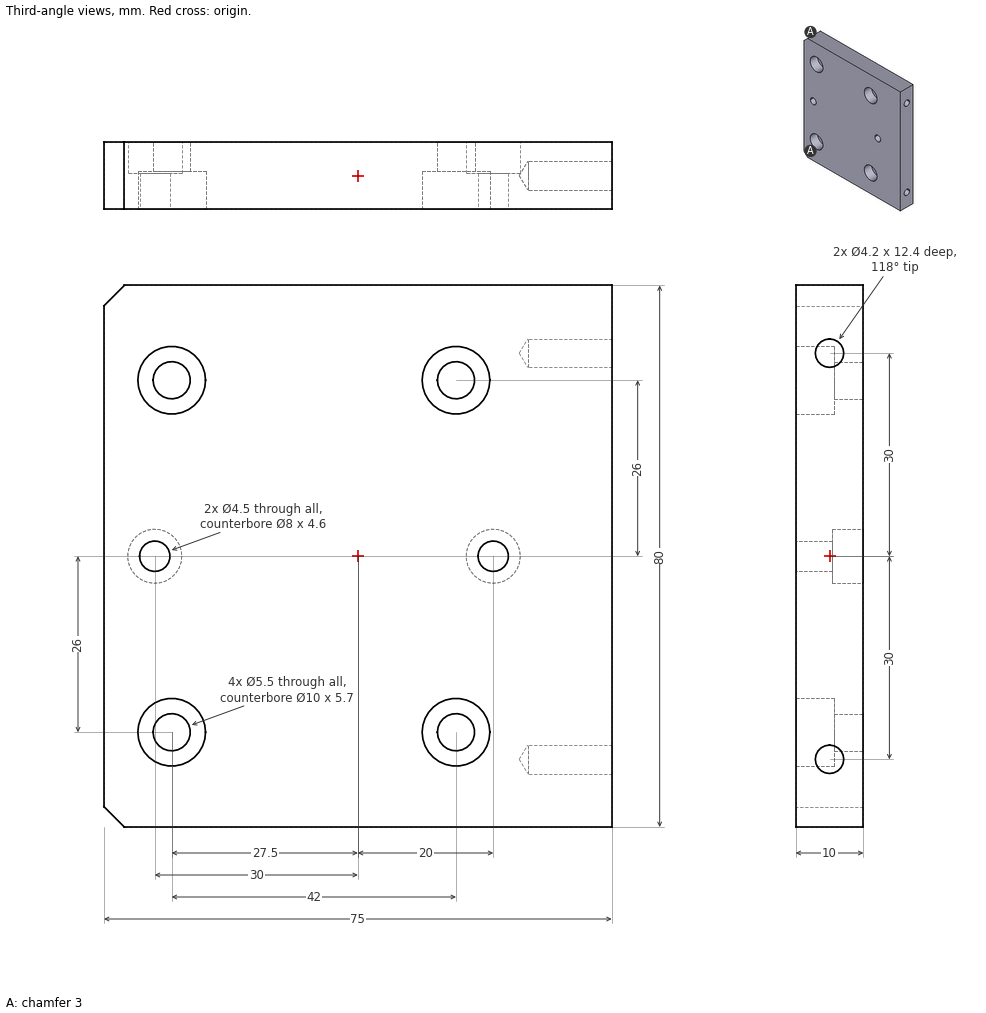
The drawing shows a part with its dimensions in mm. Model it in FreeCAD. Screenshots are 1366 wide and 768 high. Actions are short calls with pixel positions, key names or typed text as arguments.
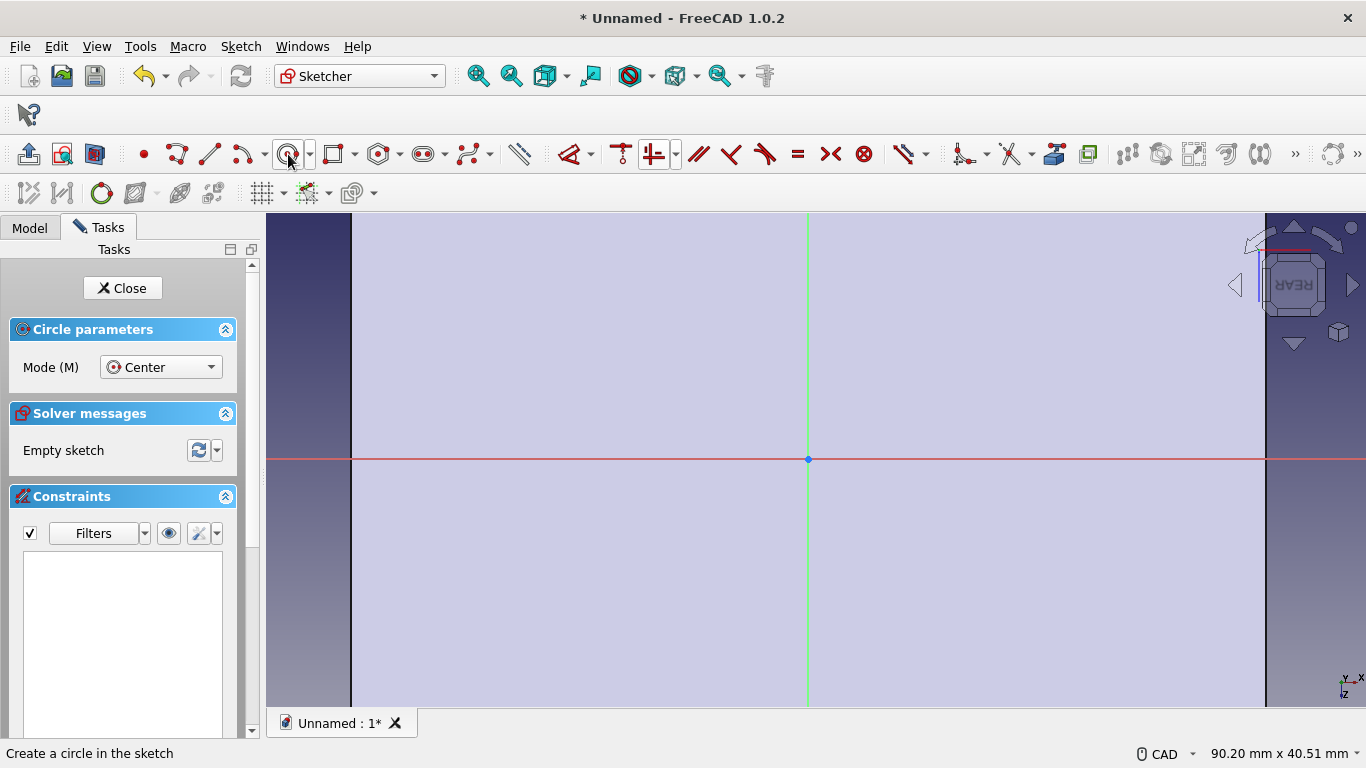
click(442, 459)
click(462, 440)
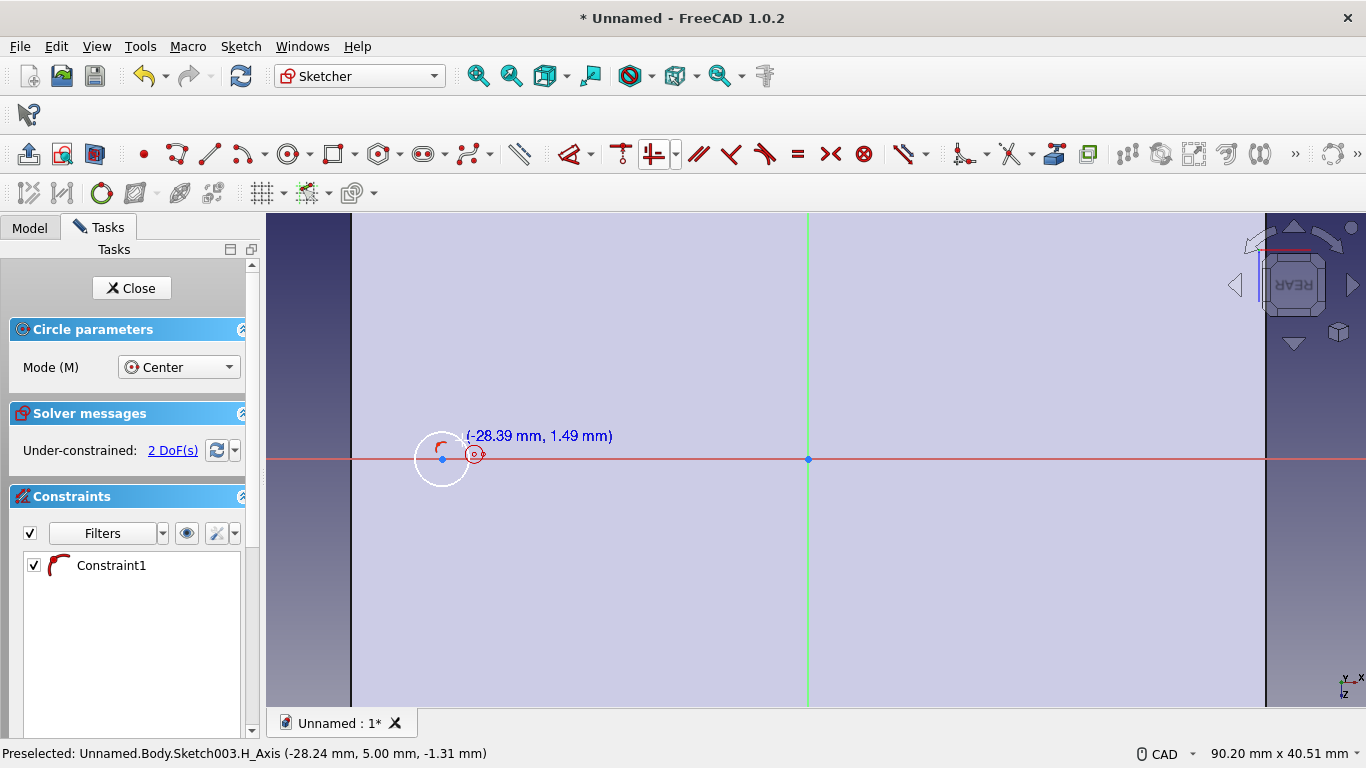
click(1052, 459)
click(1072, 440)
key(Escape)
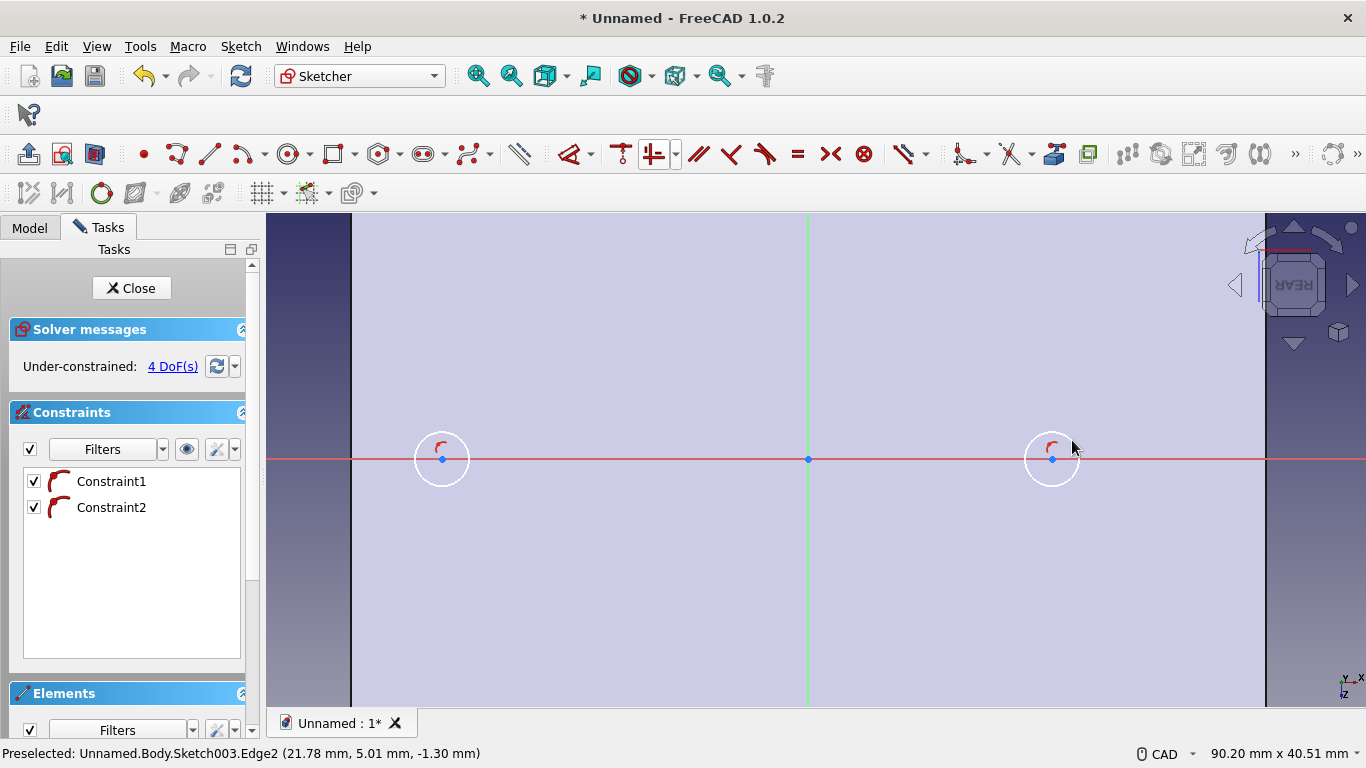
click(461, 440)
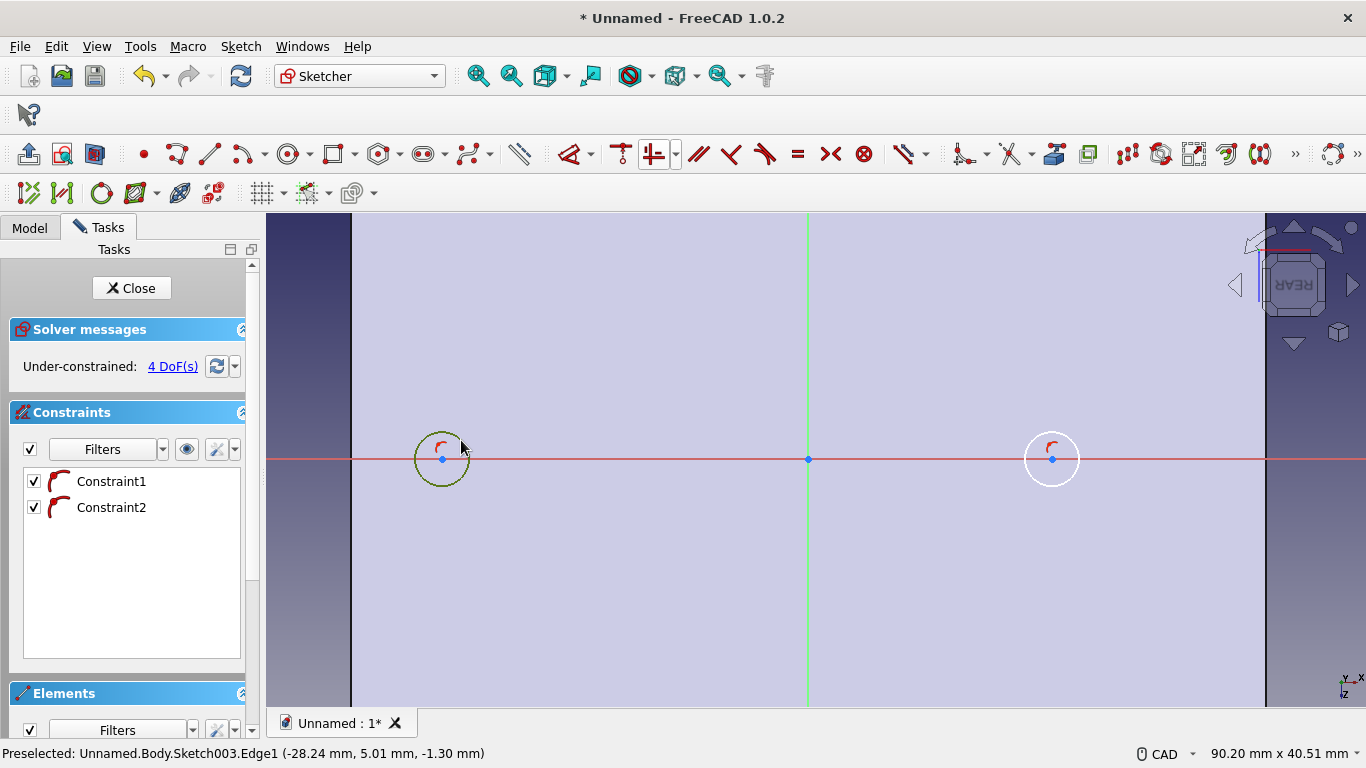
click(1071, 440)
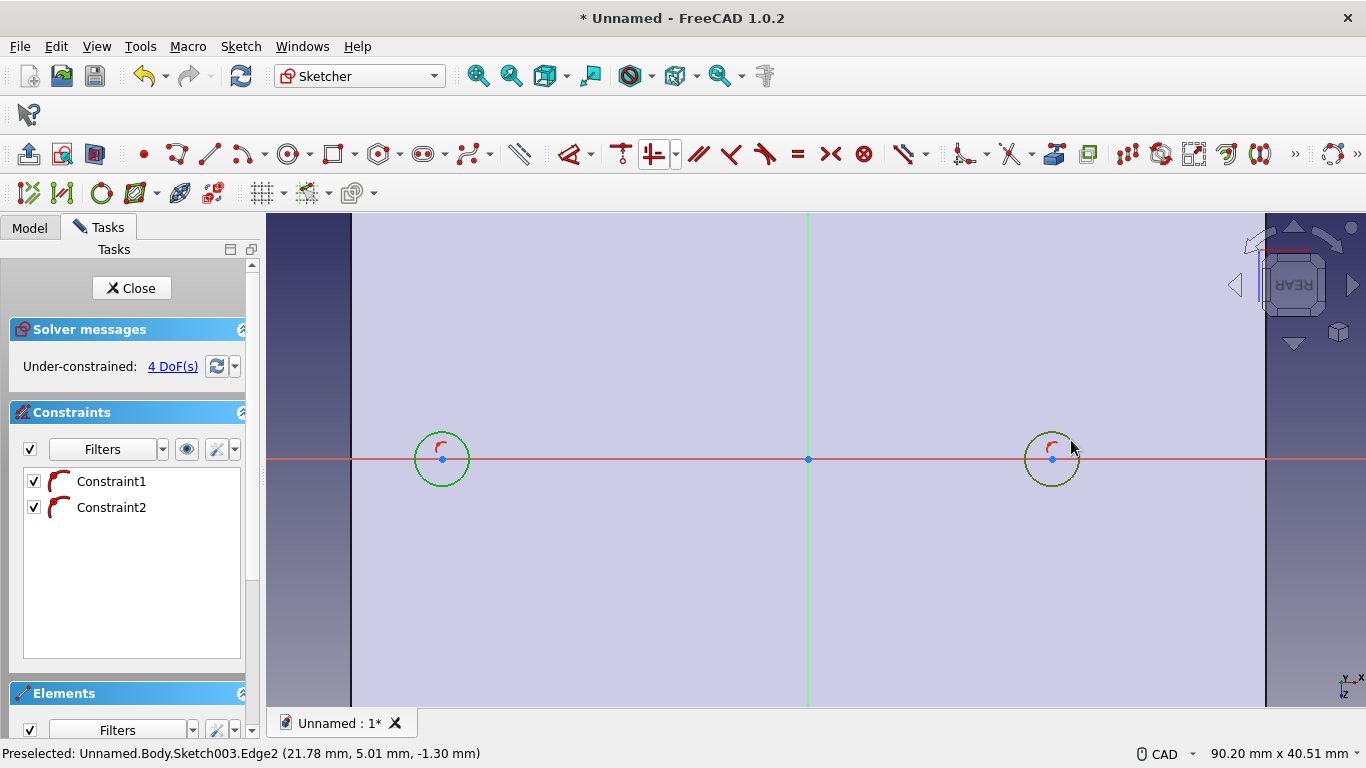
click(798, 154)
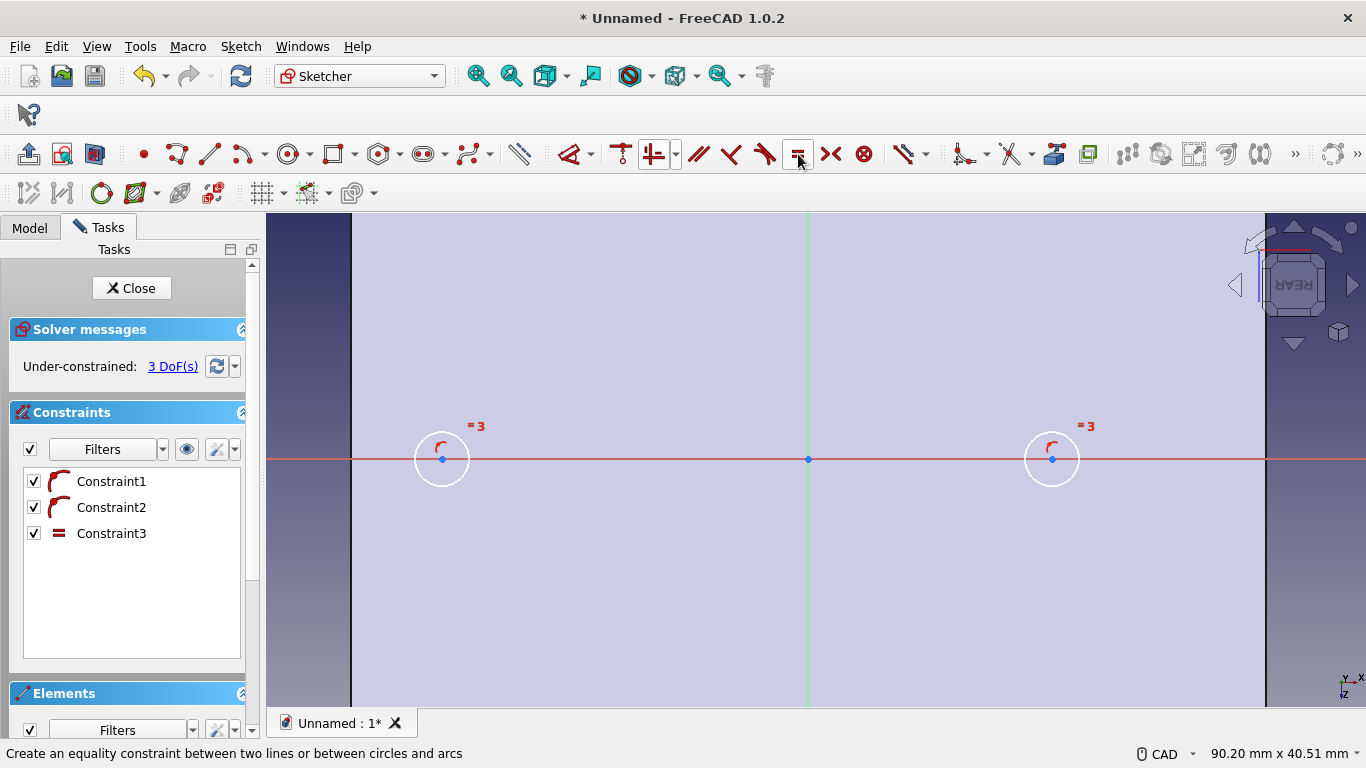
click(568, 154)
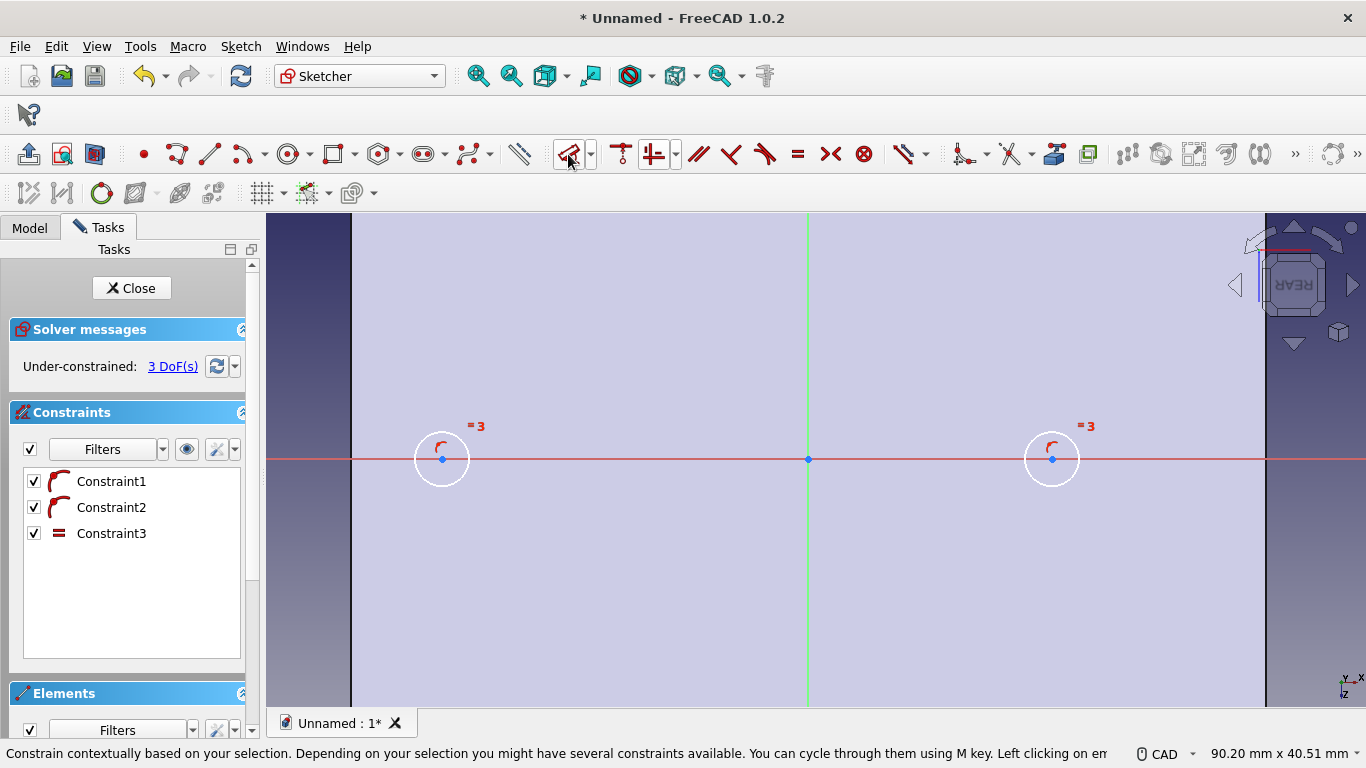
click(461, 440)
click(484, 417)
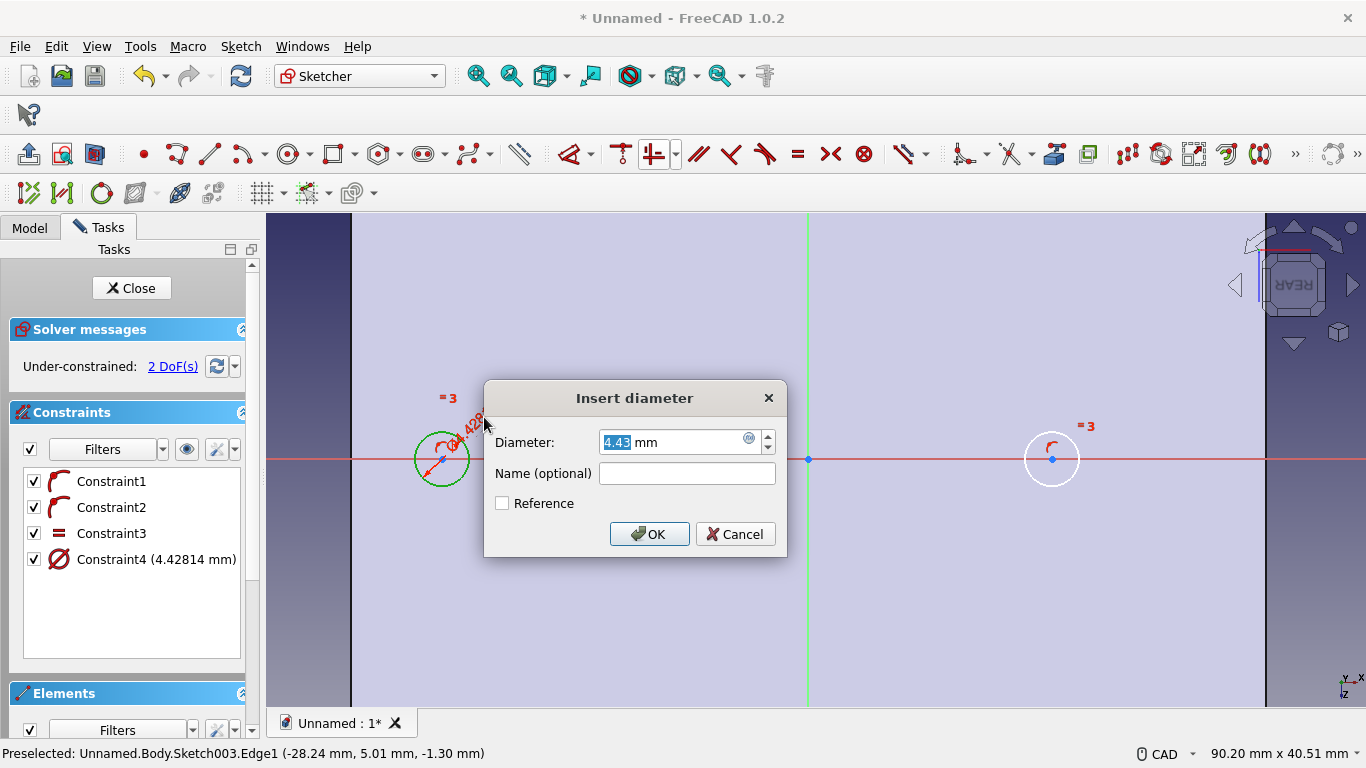
text(4.5)
key(Return)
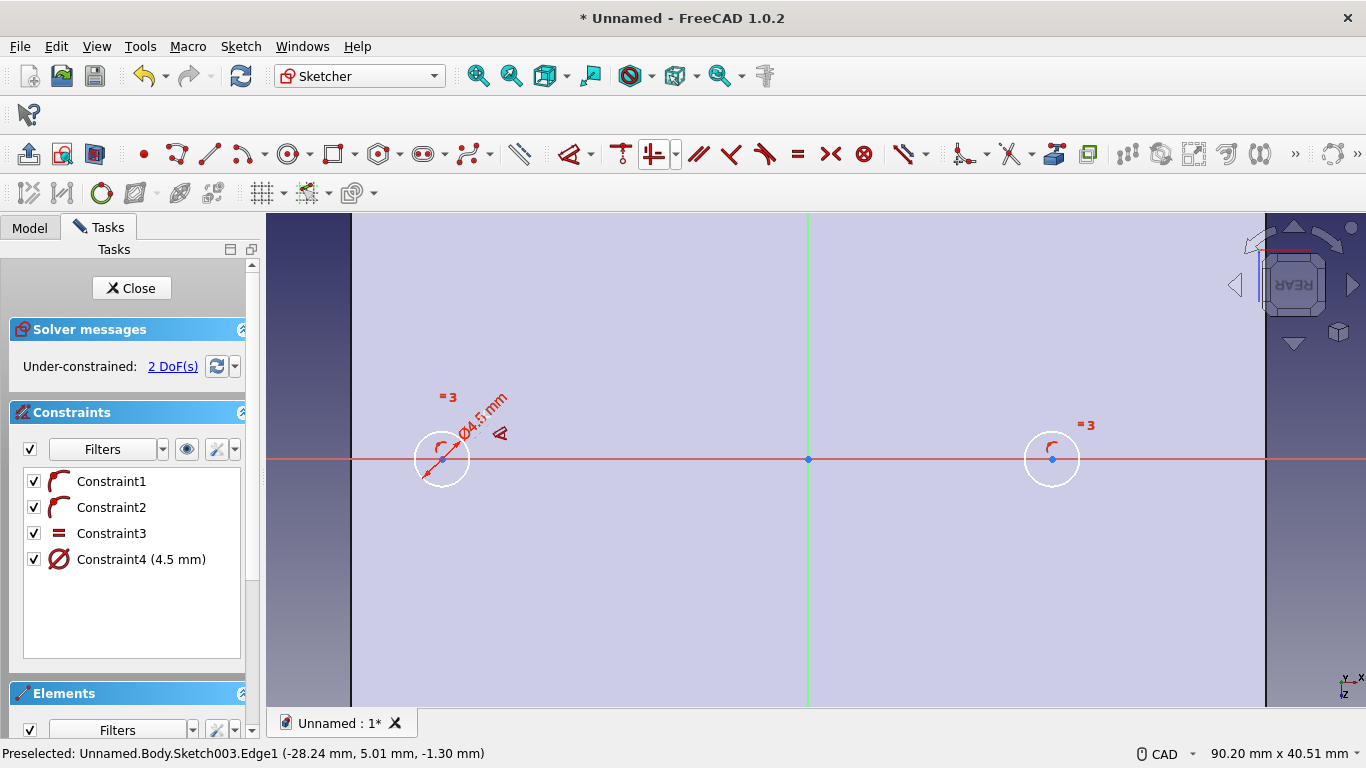
click(442, 459)
click(625, 493)